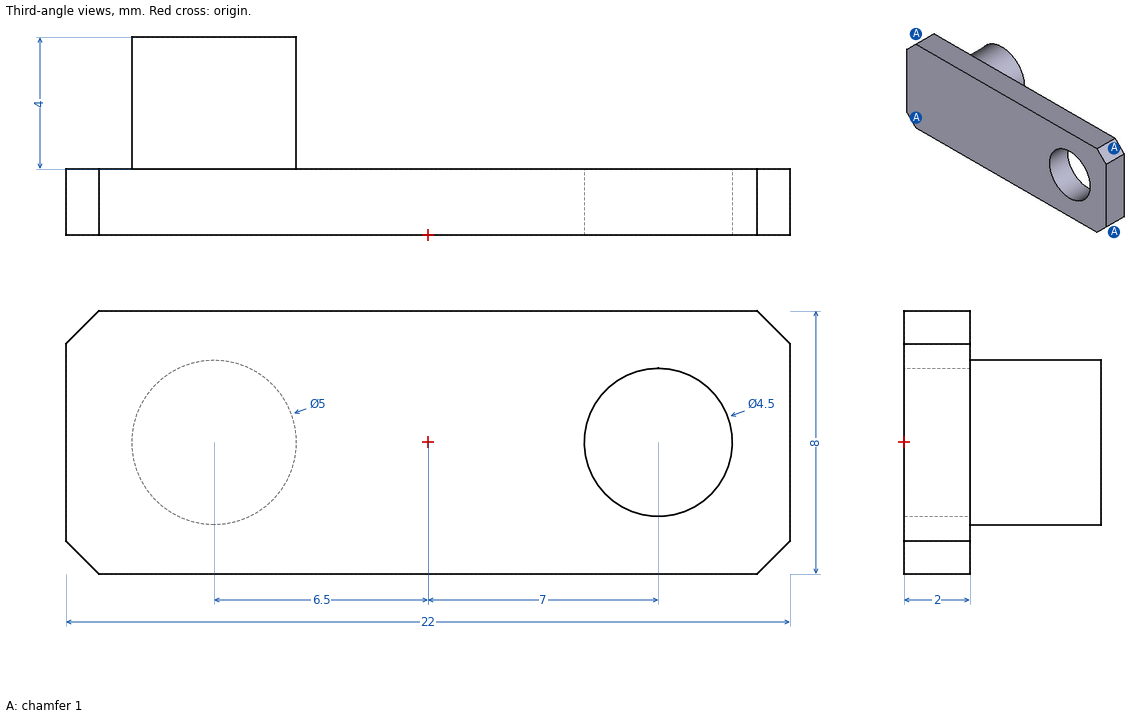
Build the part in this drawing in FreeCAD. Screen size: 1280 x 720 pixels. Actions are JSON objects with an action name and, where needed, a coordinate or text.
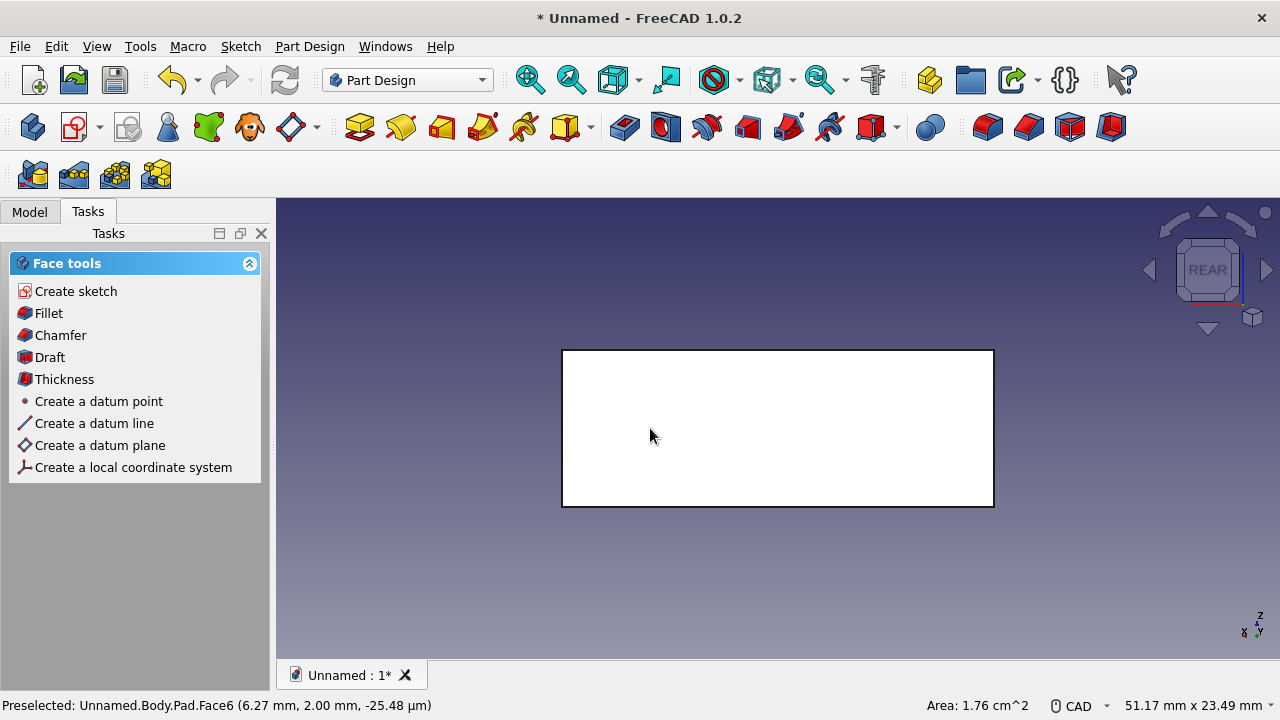
{"action": "left_click", "coordinate": [74, 128]}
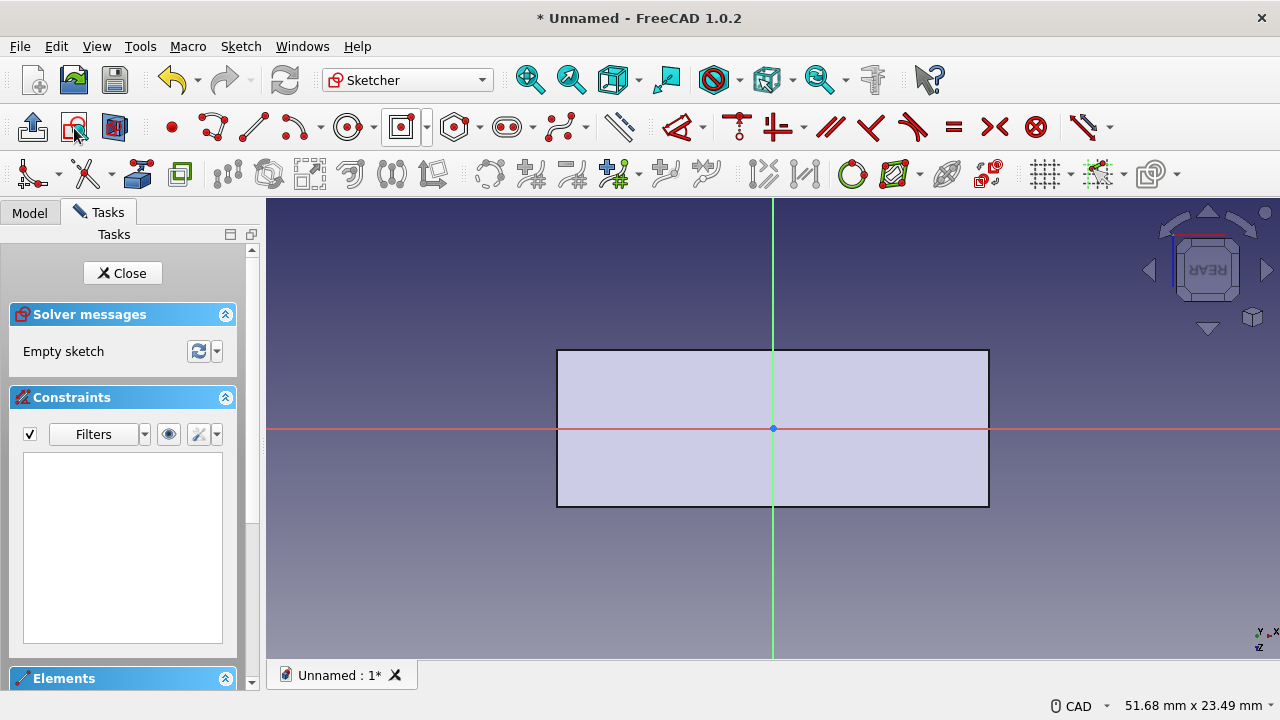
{"action": "scroll", "coordinate": [932, 428], "scroll_direction": "up", "scroll_amount": 6}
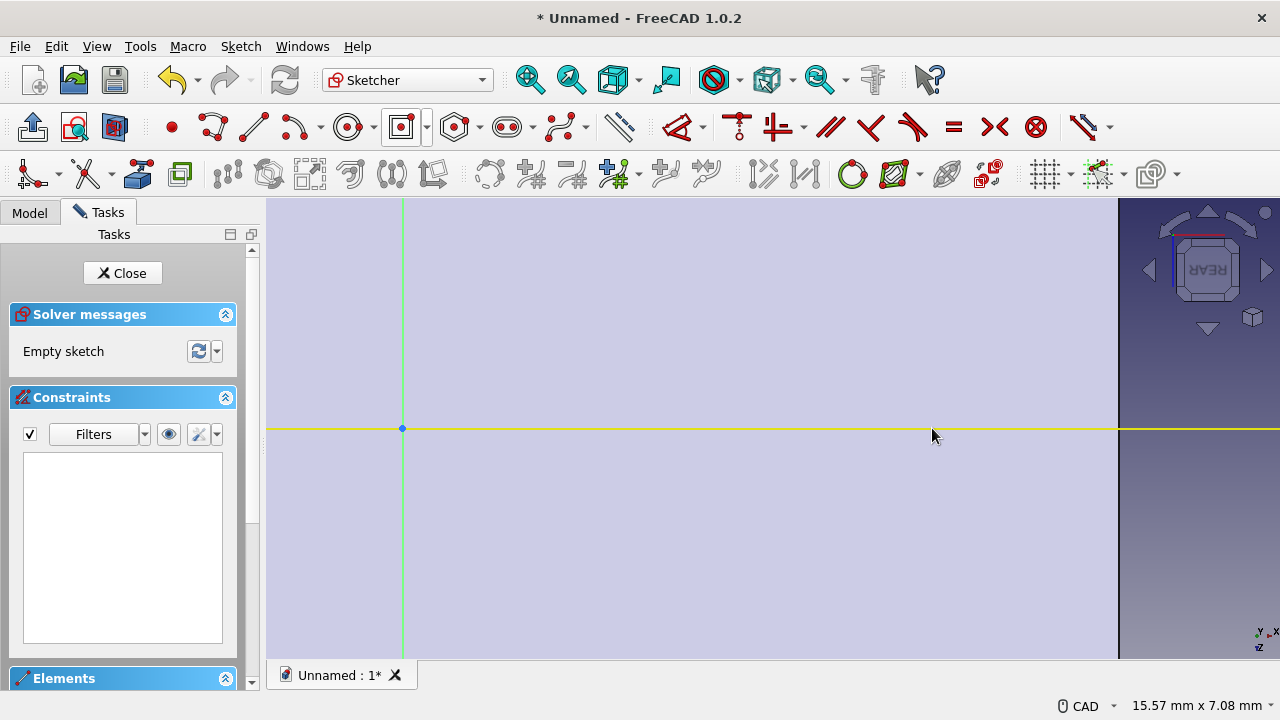
{"action": "key", "text": "g c"}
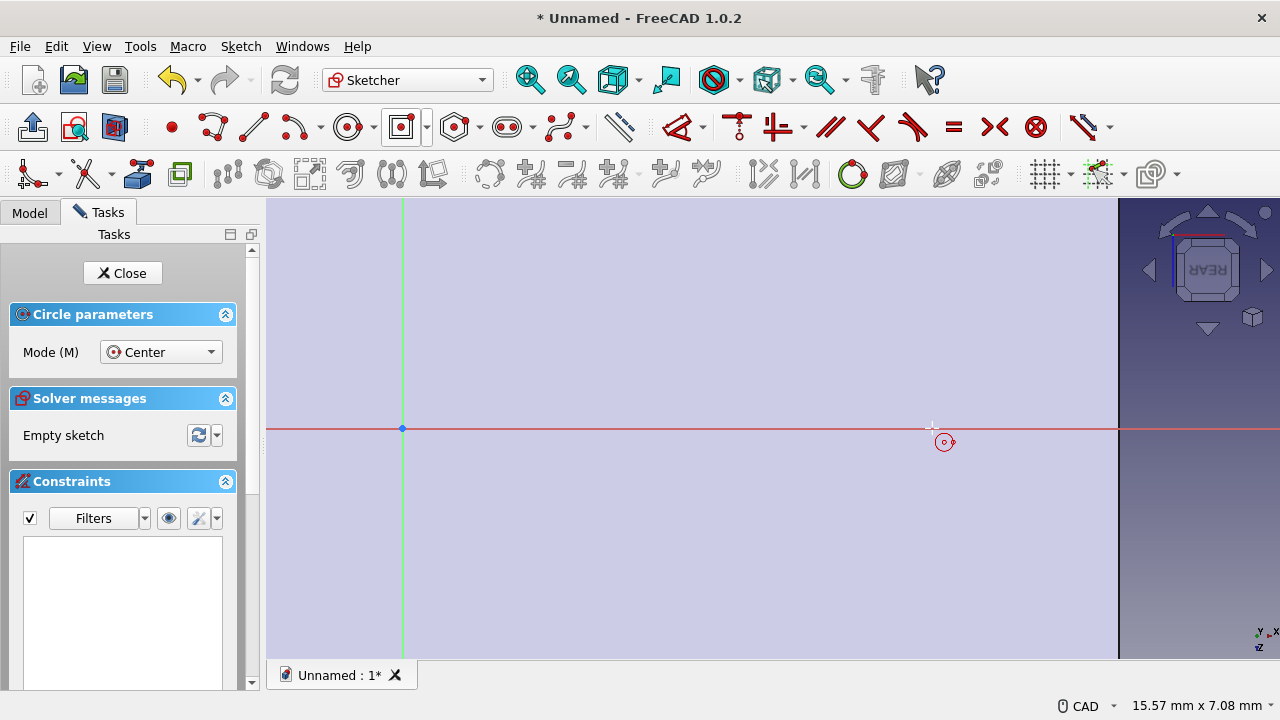
{"action": "left_click", "coordinate": [859, 428]}
{"action": "left_click", "coordinate": [962, 325]}
{"action": "key", "text": "Escape"}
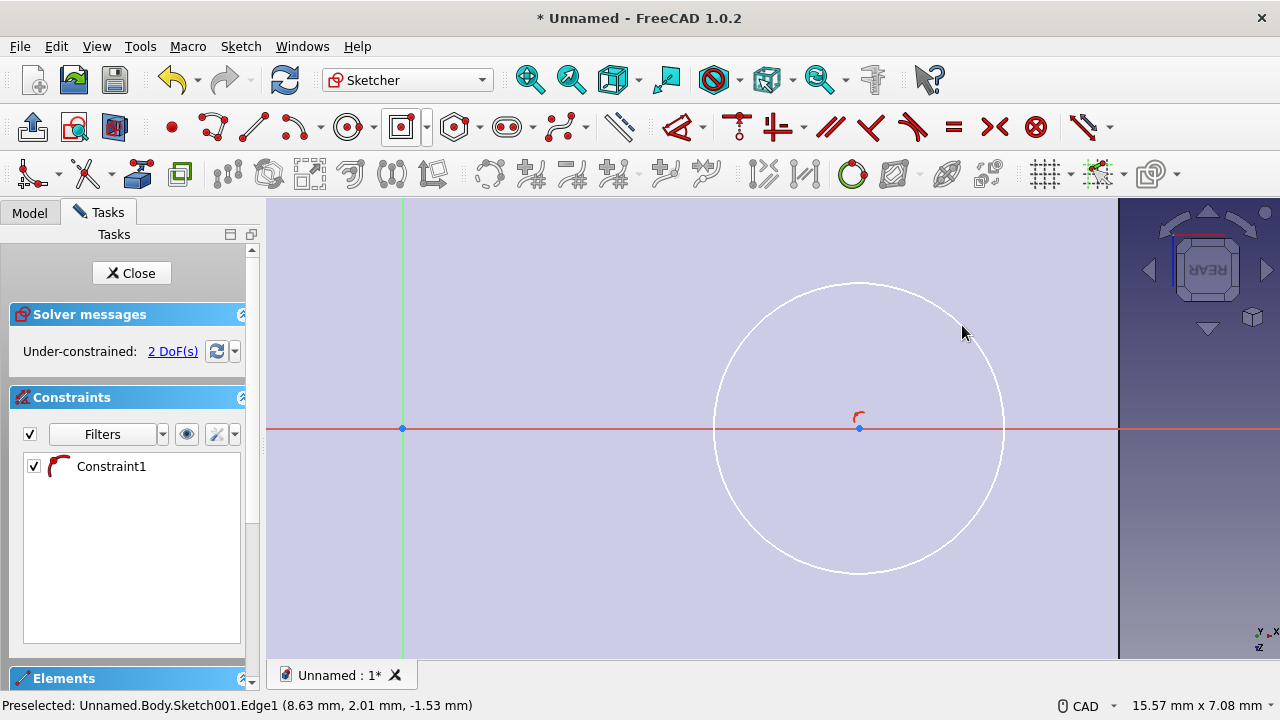
{"action": "left_click", "coordinate": [676, 128]}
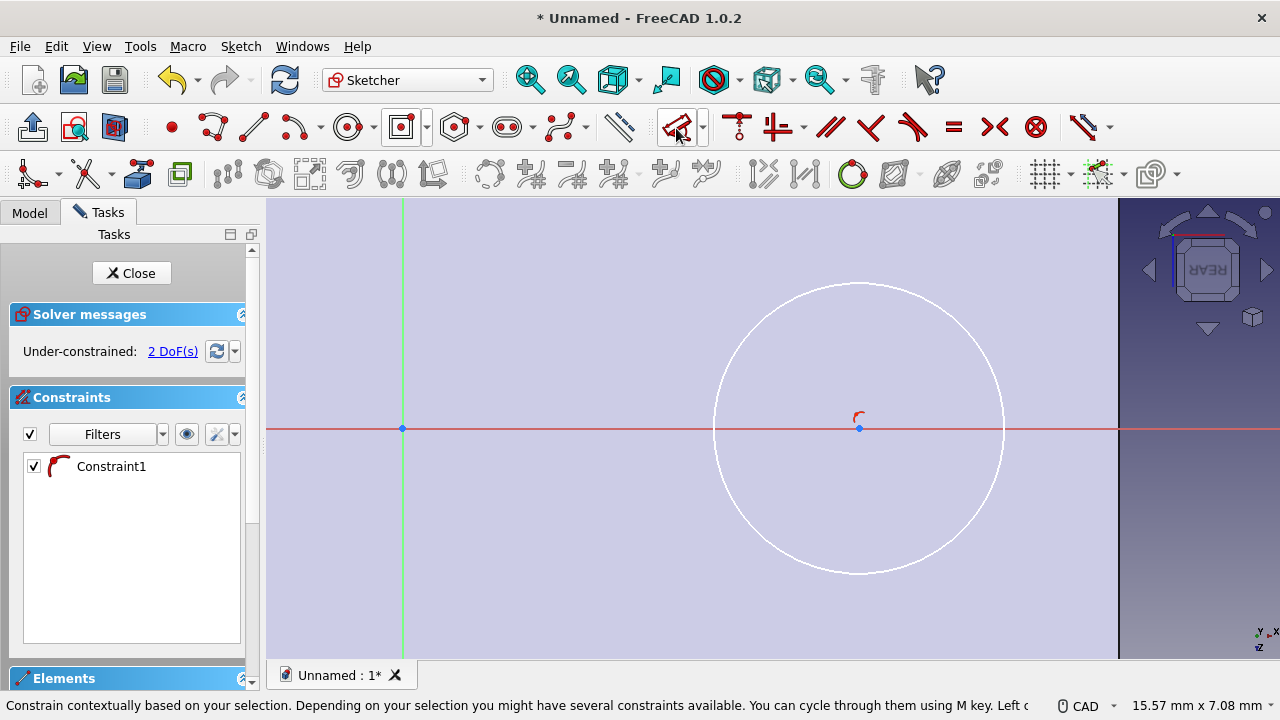
{"action": "left_click", "coordinate": [961, 325]}
{"action": "left_click", "coordinate": [983, 302]}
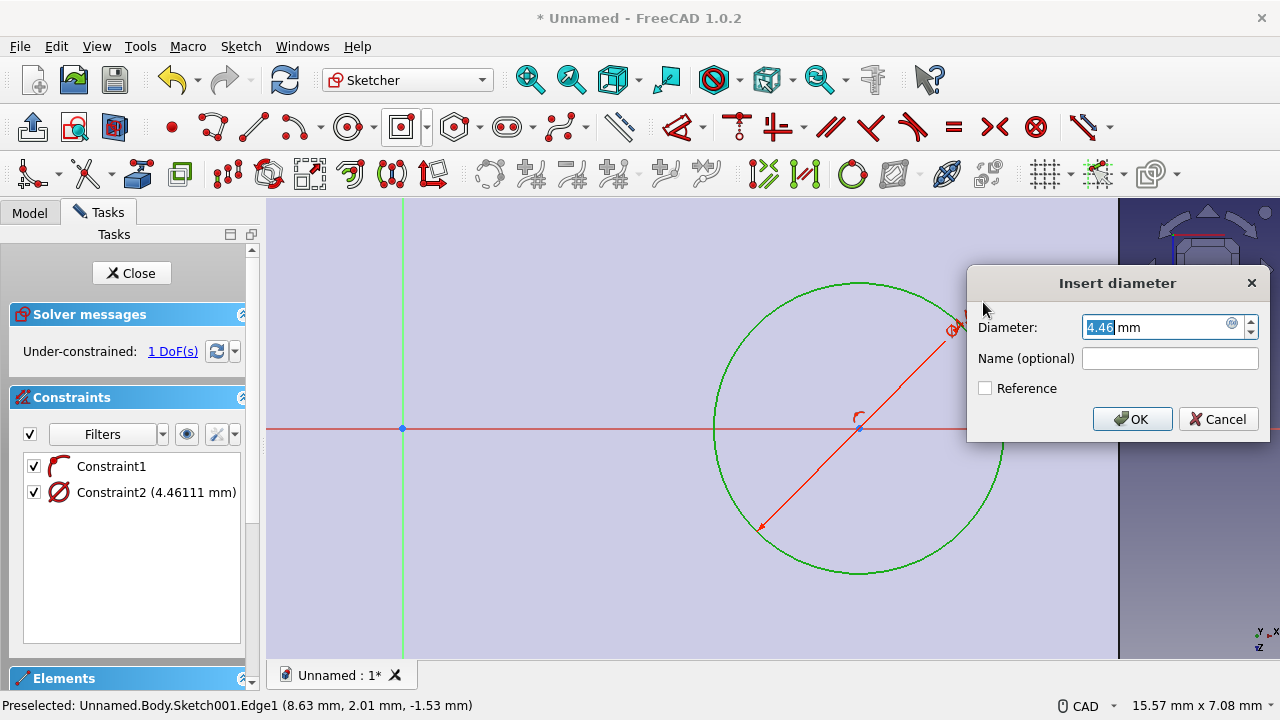
{"action": "type", "text": "4.5"}
{"action": "key", "text": "Return"}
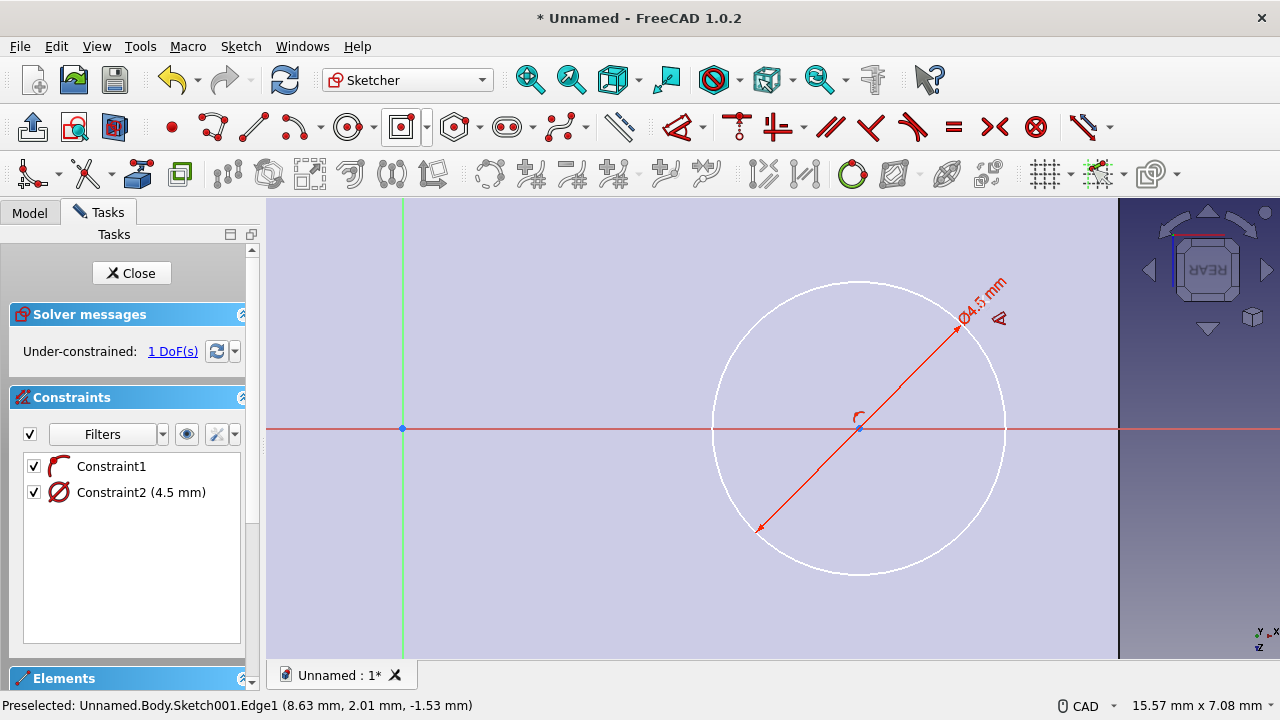
{"action": "left_click", "coordinate": [859, 428]}
{"action": "left_click", "coordinate": [631, 462]}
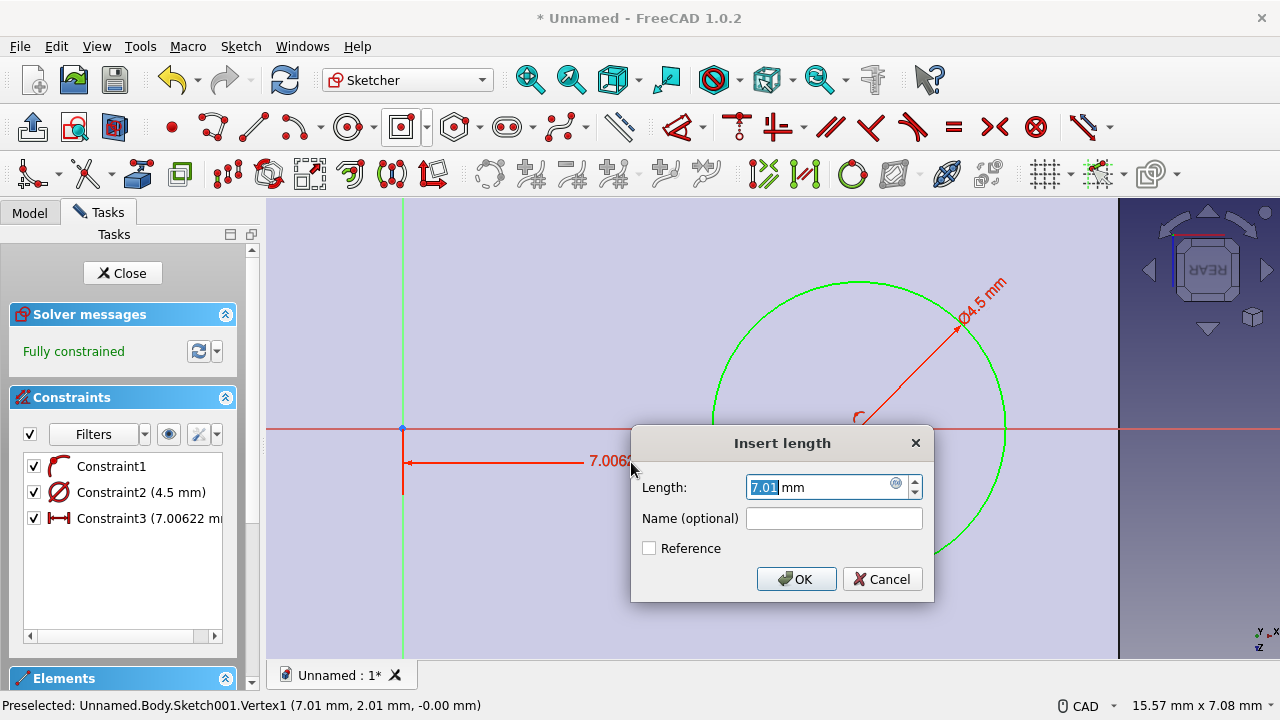
{"action": "type", "text": "7"}
{"action": "key", "text": "Return"}
{"action": "key", "text": "Escape"}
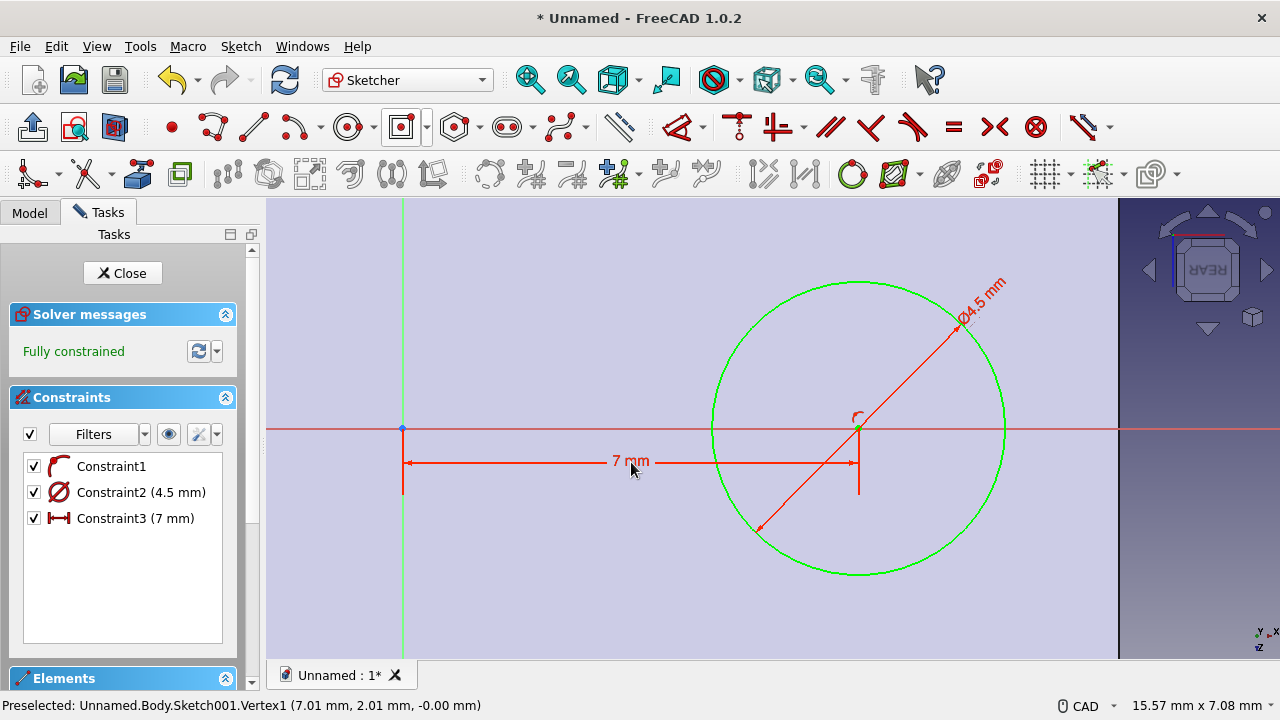
{"action": "left_click", "coordinate": [123, 273]}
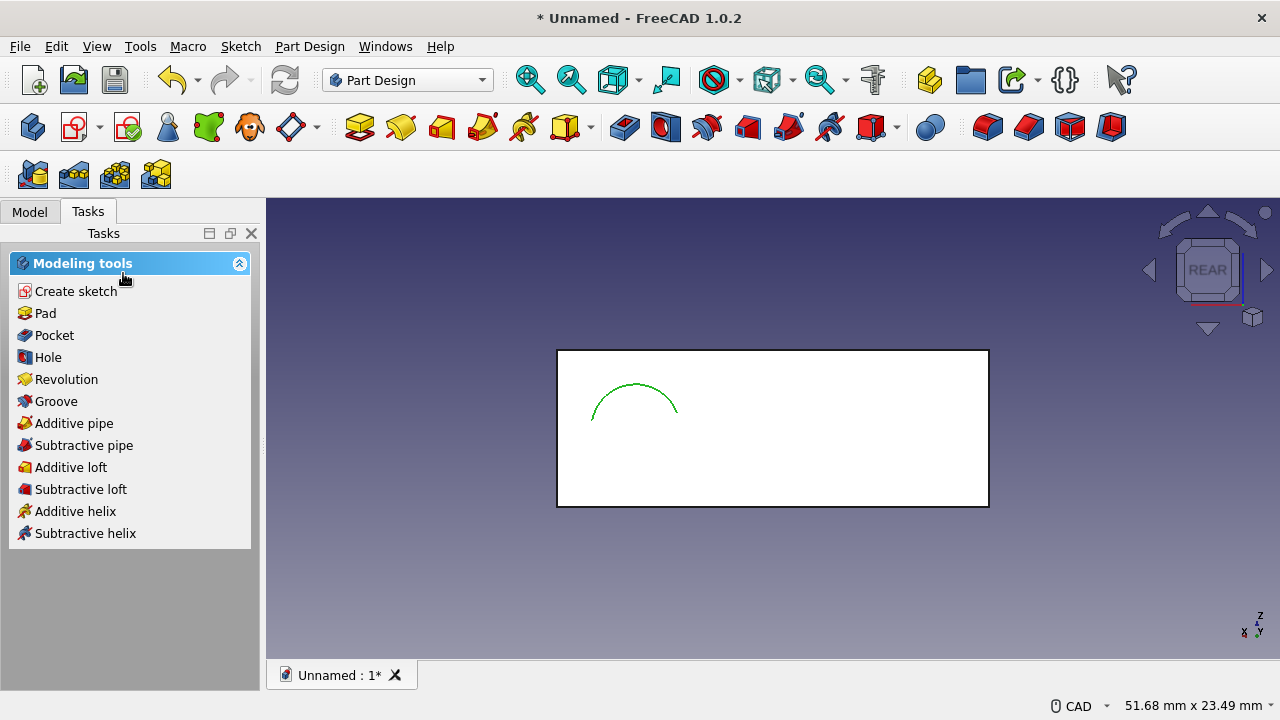
{"action": "left_click", "coordinate": [625, 128]}